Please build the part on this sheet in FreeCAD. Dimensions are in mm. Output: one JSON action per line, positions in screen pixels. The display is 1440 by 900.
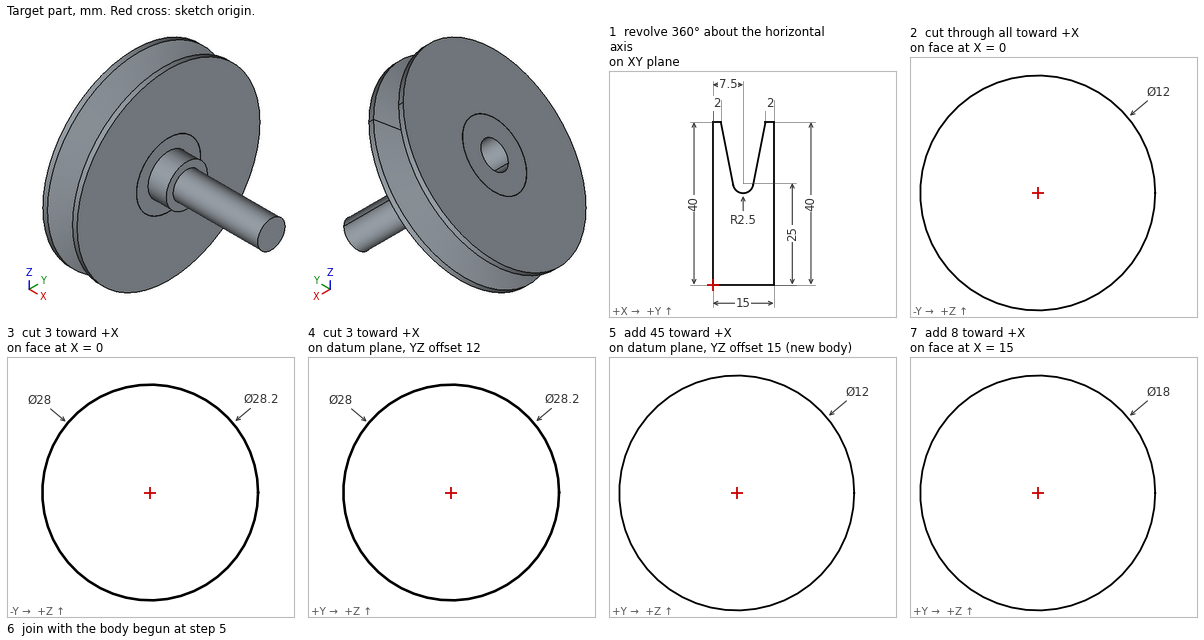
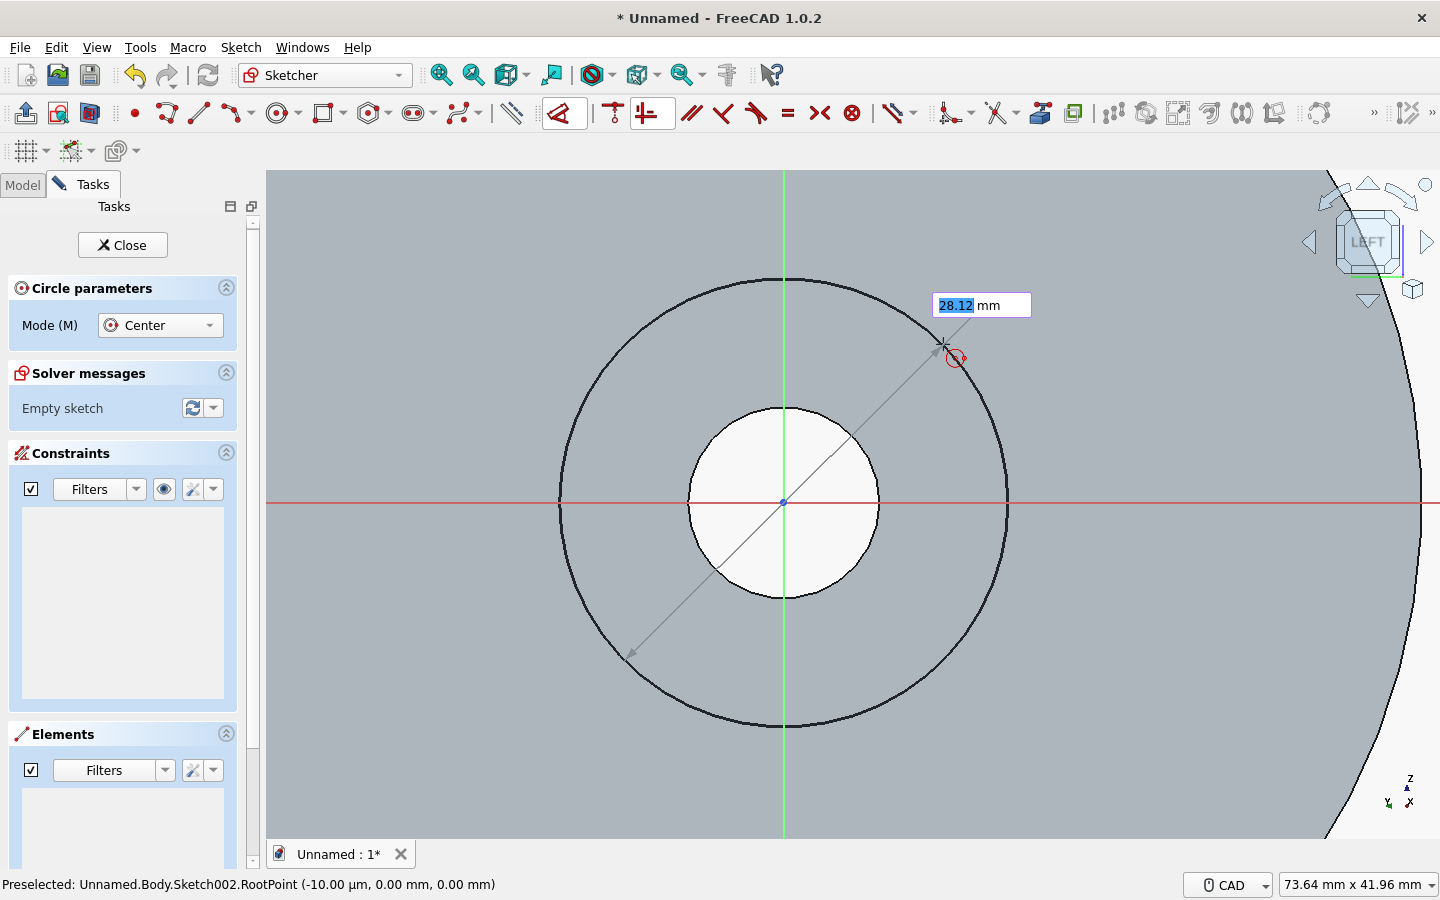
{"action": "type", "text": "28.2"}
{"action": "key", "text": "Return"}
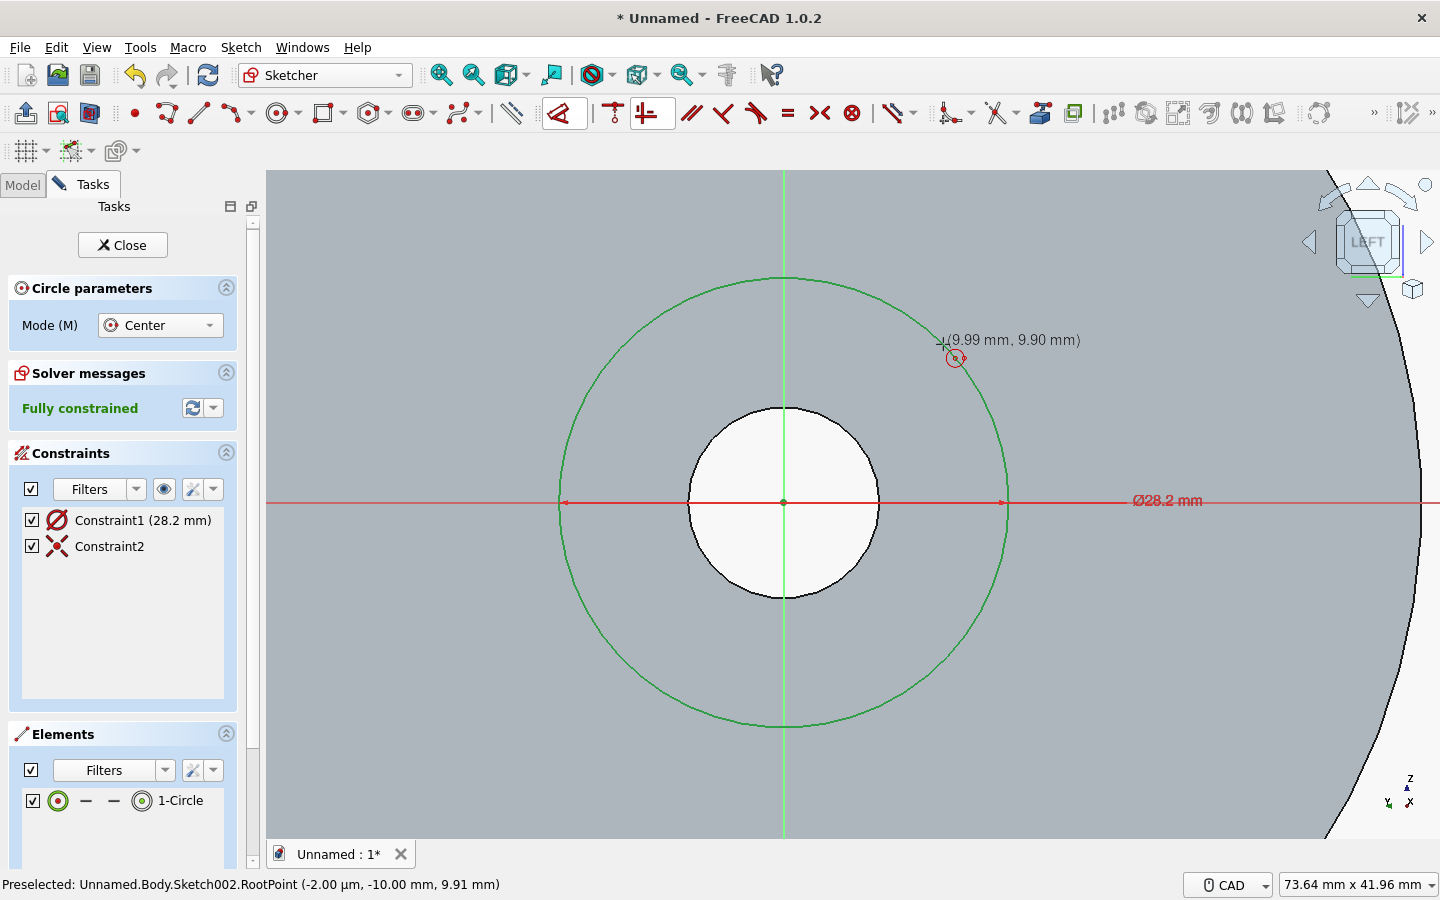
{"action": "left_click", "coordinate": [784, 503]}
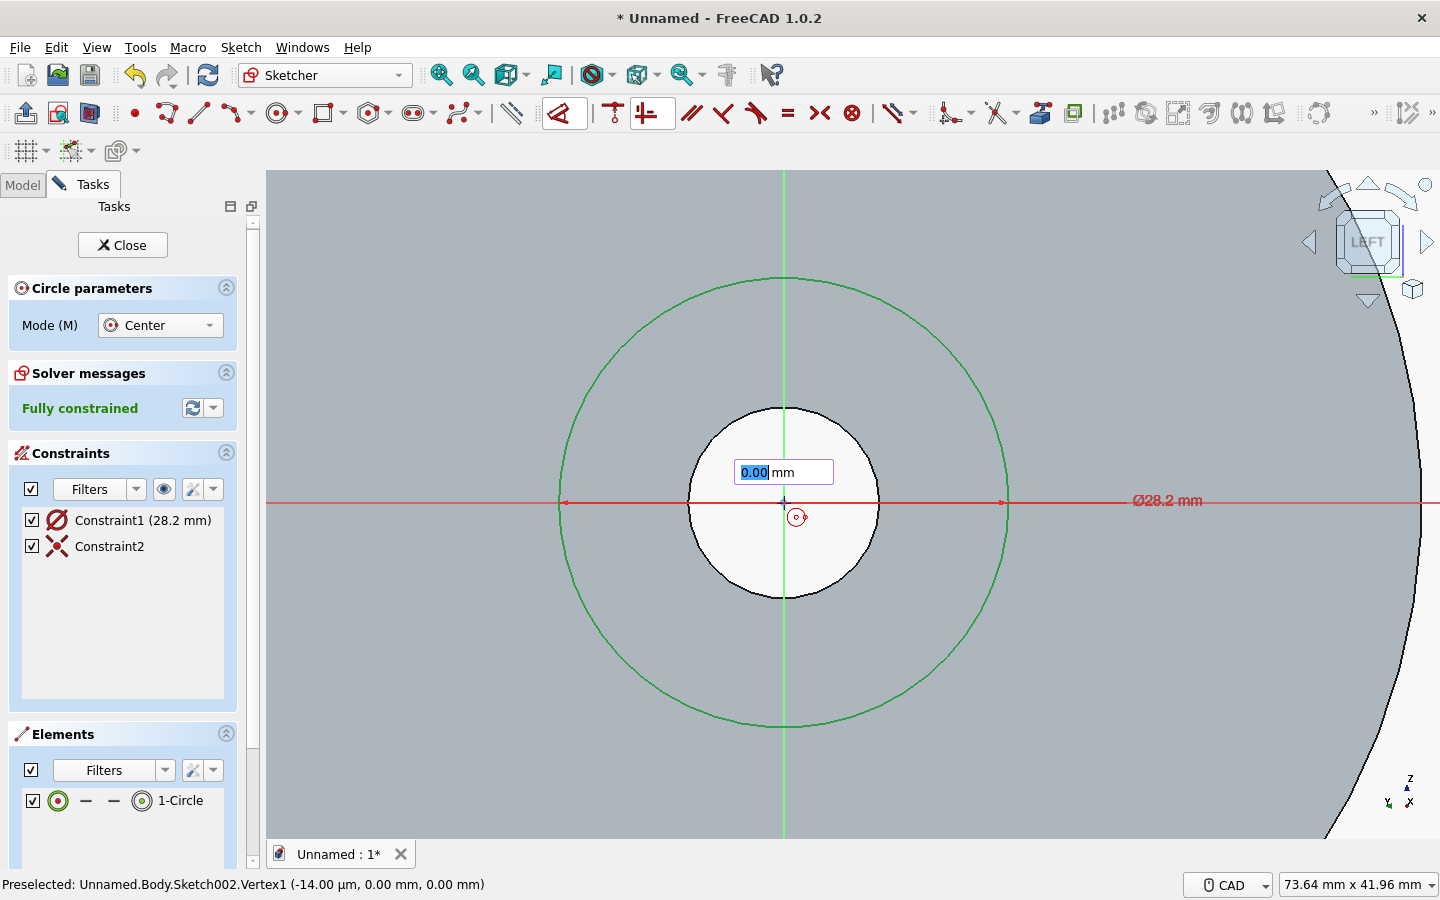
{"action": "scroll", "coordinate": [942, 345], "scroll_direction": "up", "scroll_amount": 12}
{"action": "mouse_move", "coordinate": [932, 342]}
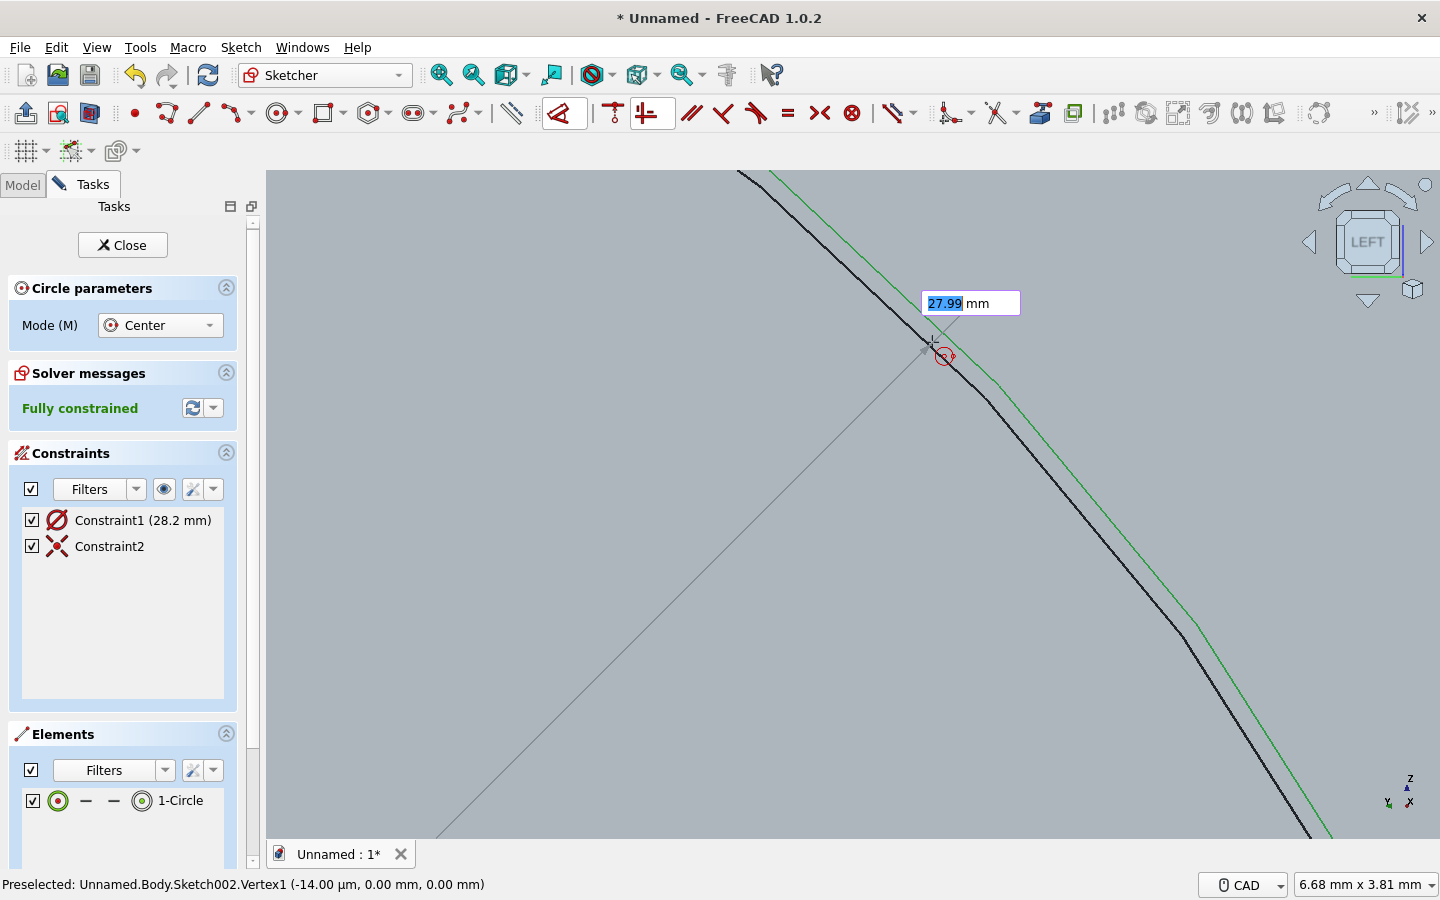
{"action": "type", "text": "28"}
{"action": "key", "text": "Return"}
{"action": "key", "text": "Escape"}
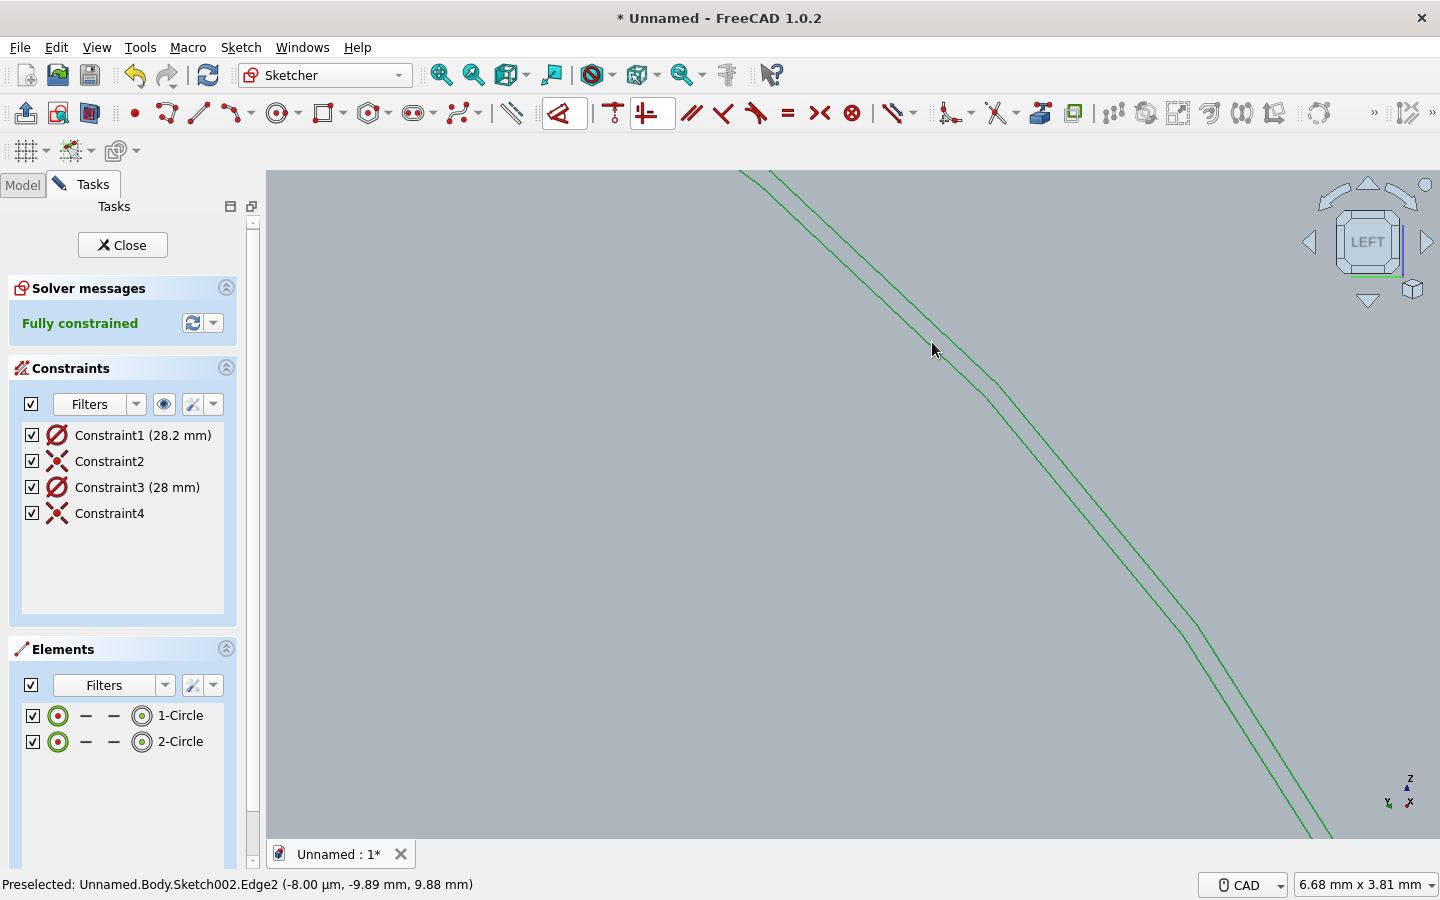
{"action": "left_click", "coordinate": [123, 245]}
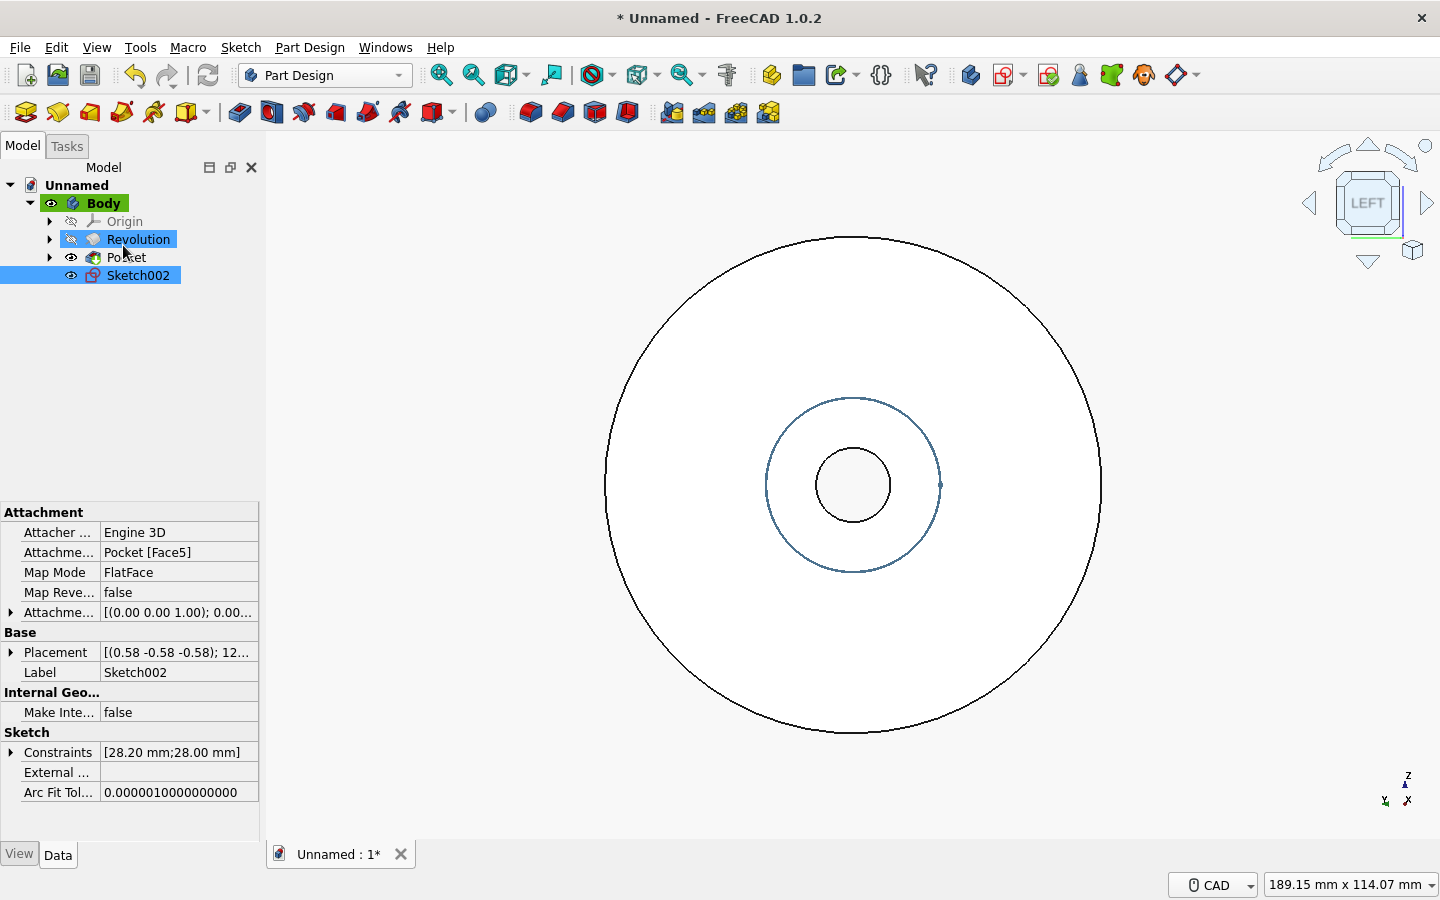
{"action": "left_click", "coordinate": [240, 112]}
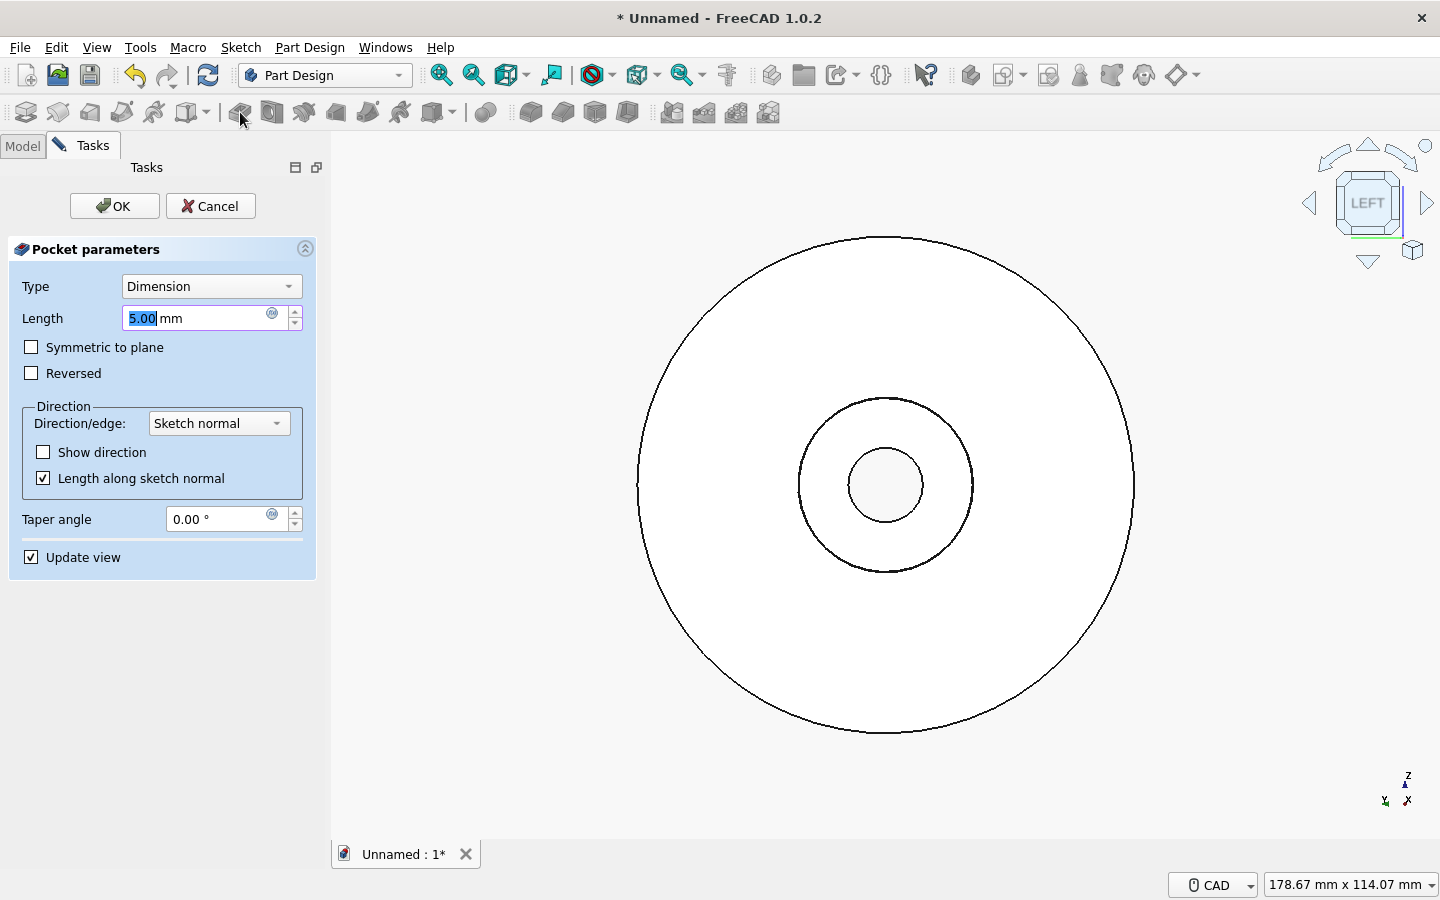
{"action": "type", "text": "3"}
{"action": "key", "text": "Tab"}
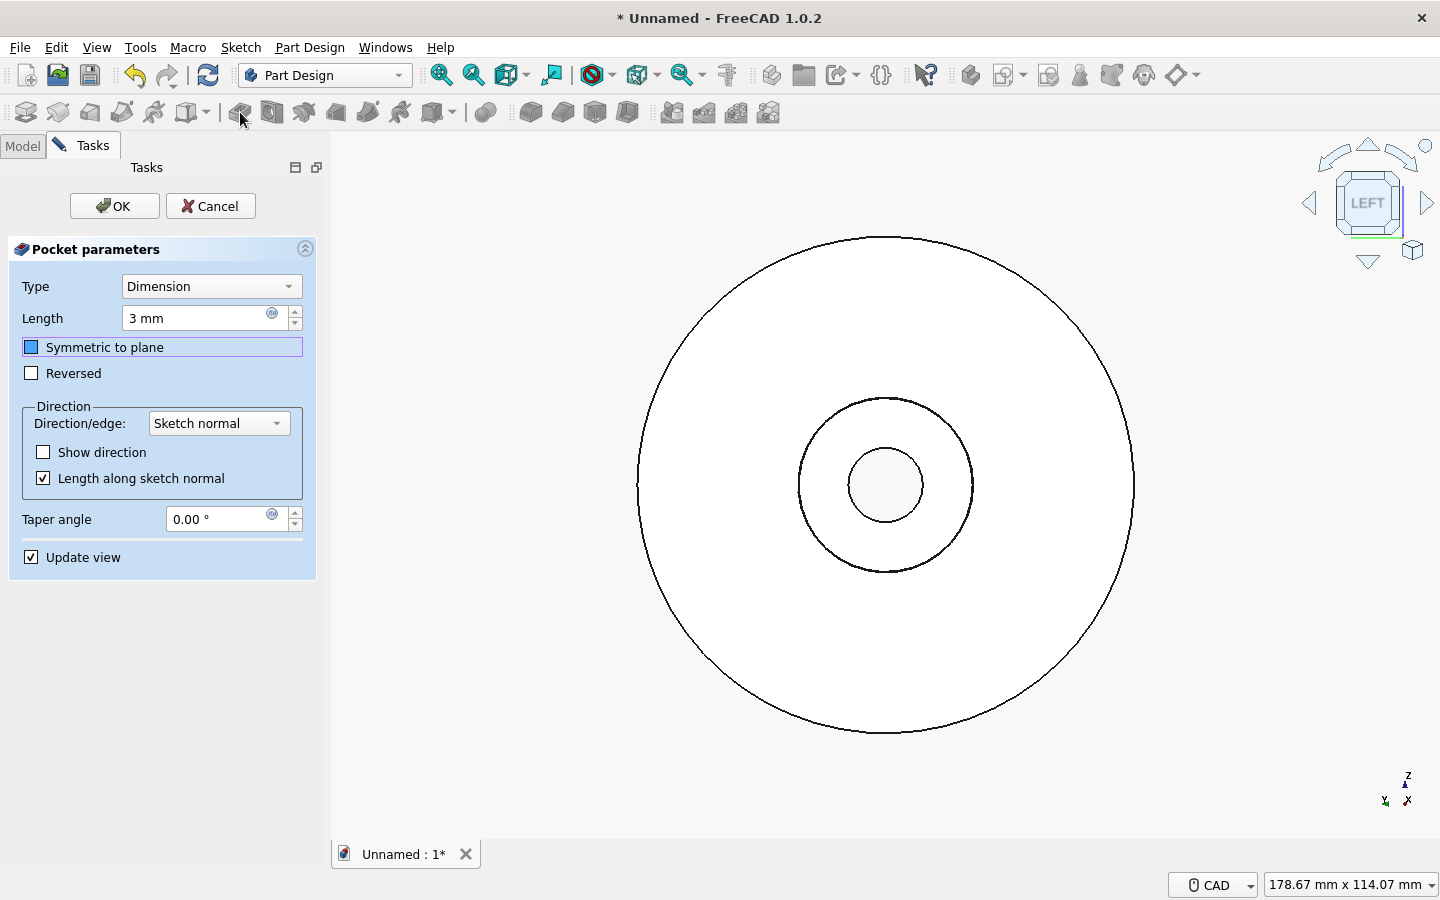
{"action": "left_click", "coordinate": [115, 206]}